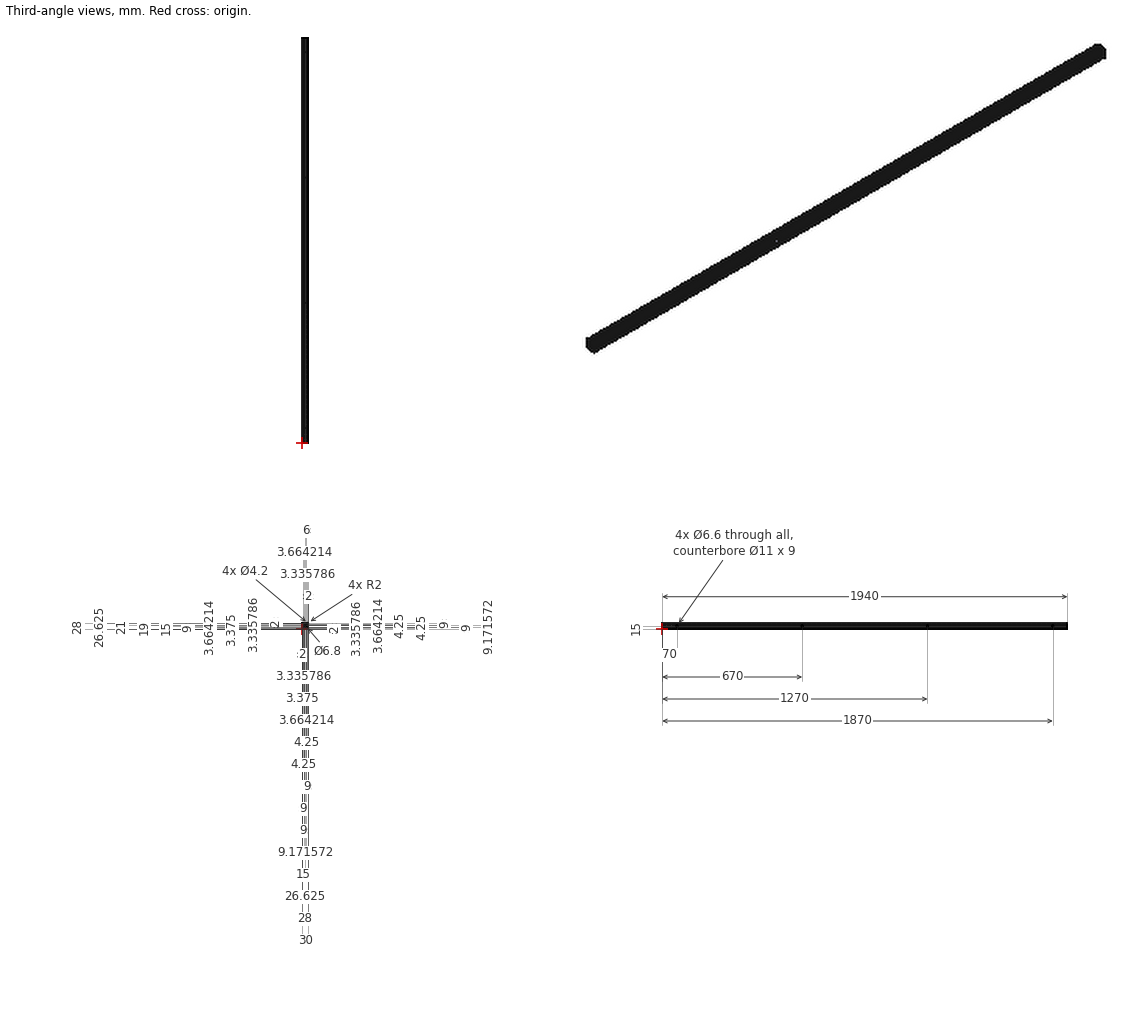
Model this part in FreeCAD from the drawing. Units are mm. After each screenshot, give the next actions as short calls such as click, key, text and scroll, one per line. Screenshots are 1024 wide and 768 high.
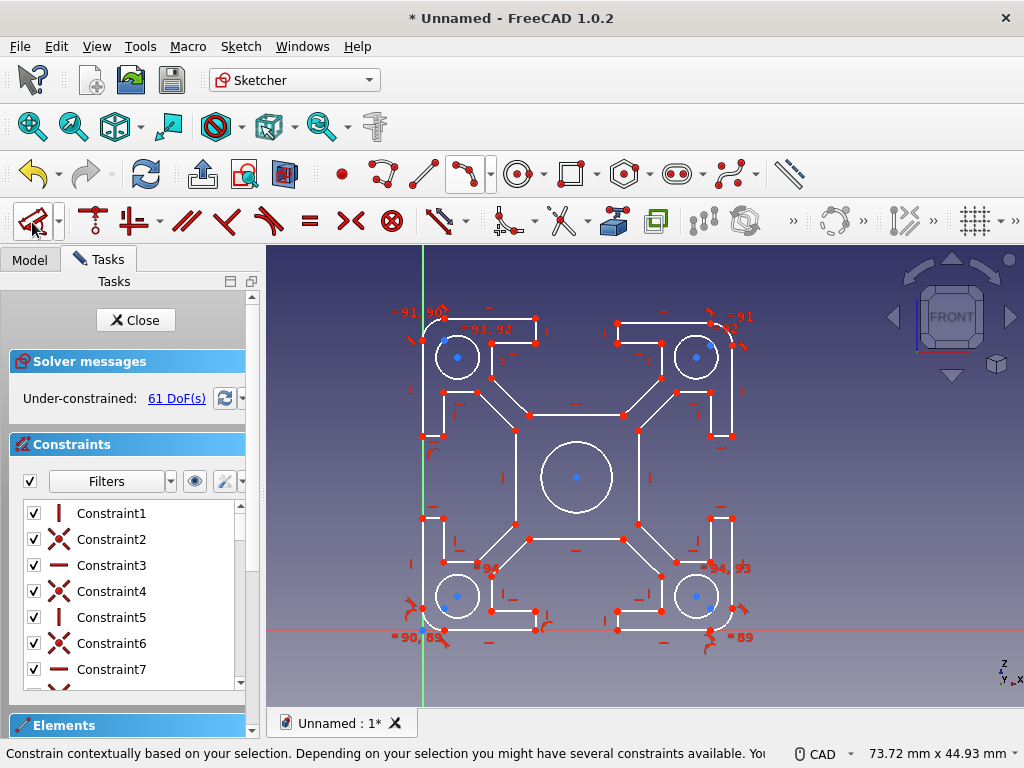
scroll(721, 628, up, 4)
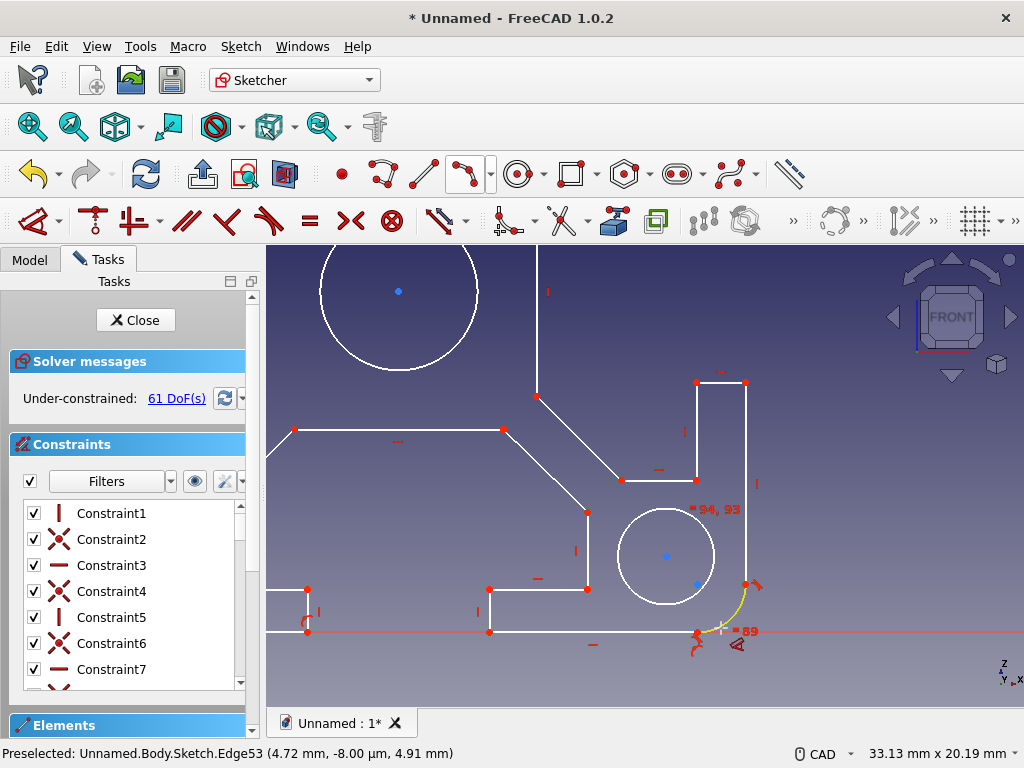
click(719, 627)
click(733, 656)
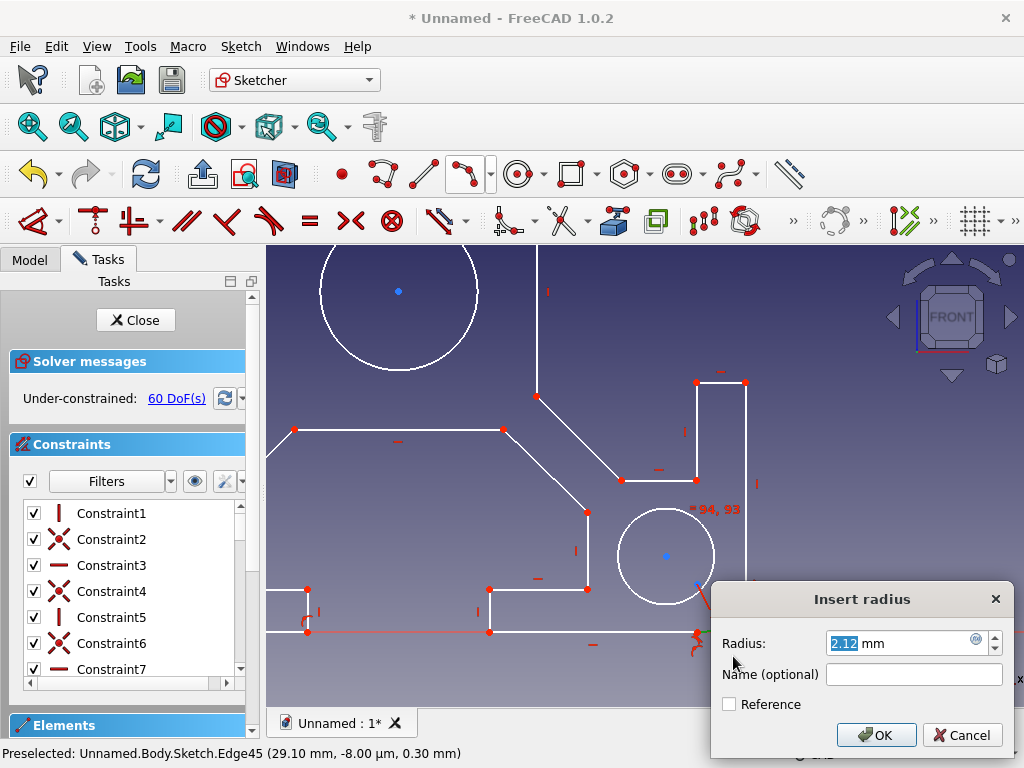
text(2)
key(Return)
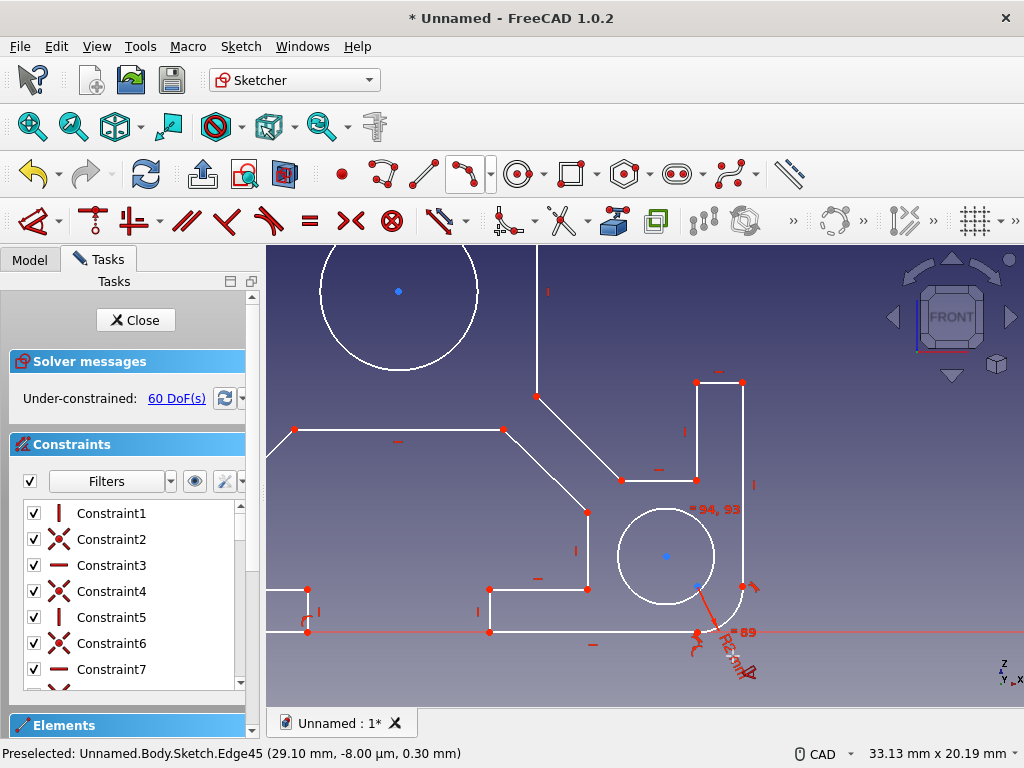
scroll(721, 628, down, 4)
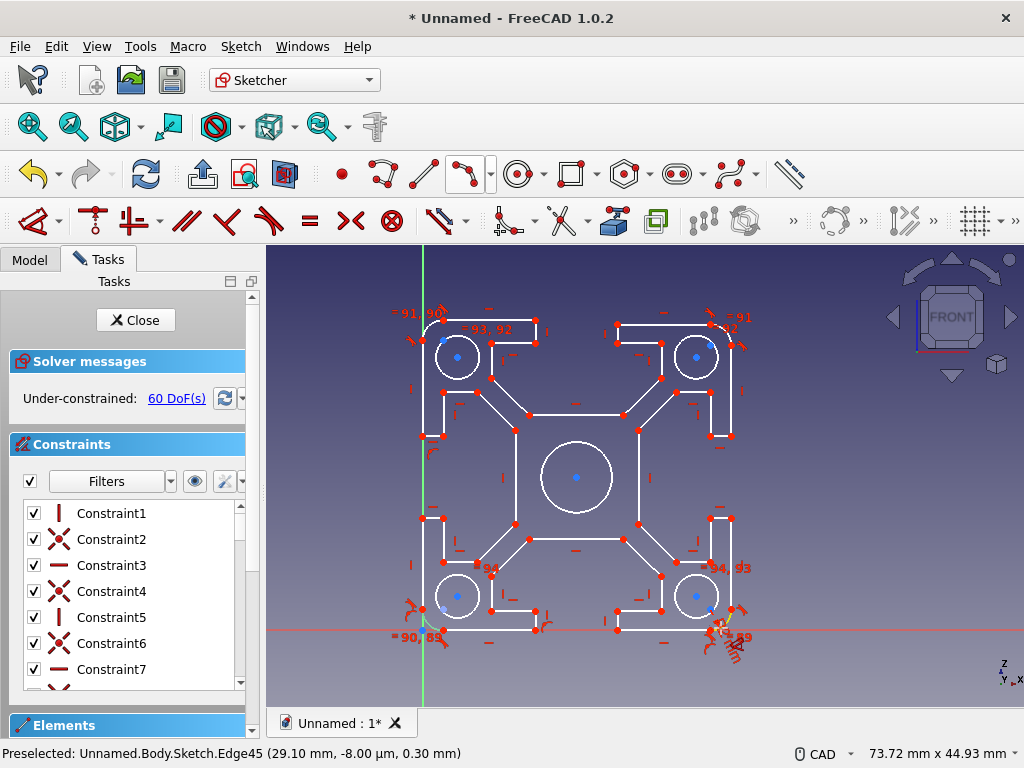
click(681, 342)
click(681, 306)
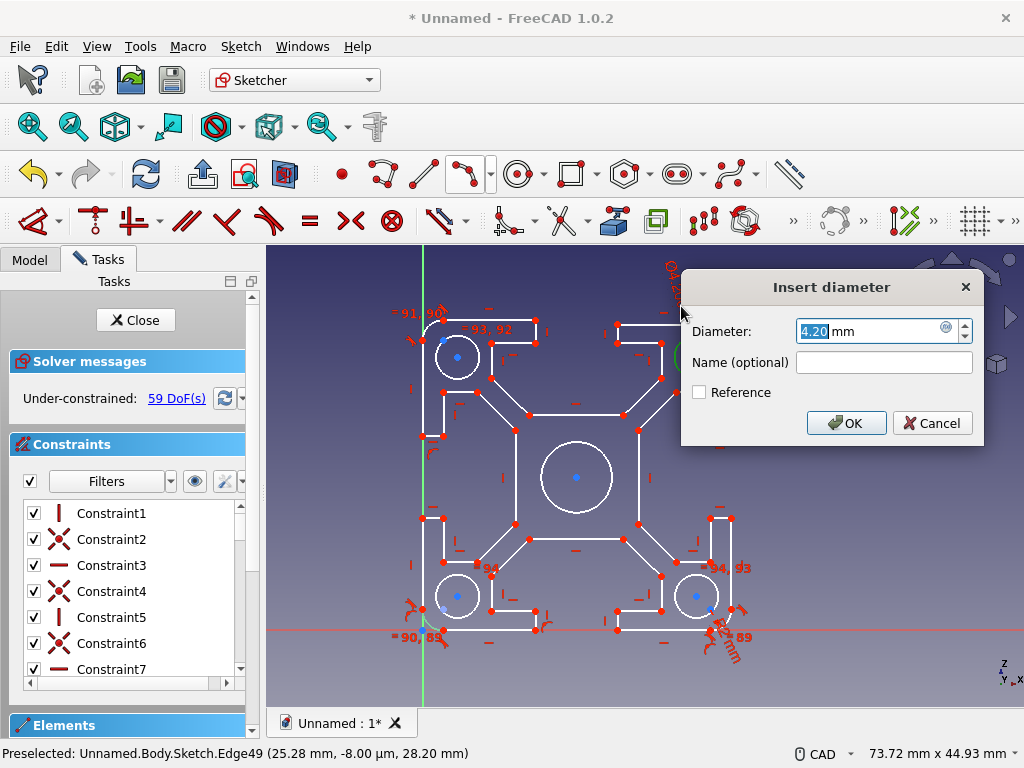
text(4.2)
key(Return)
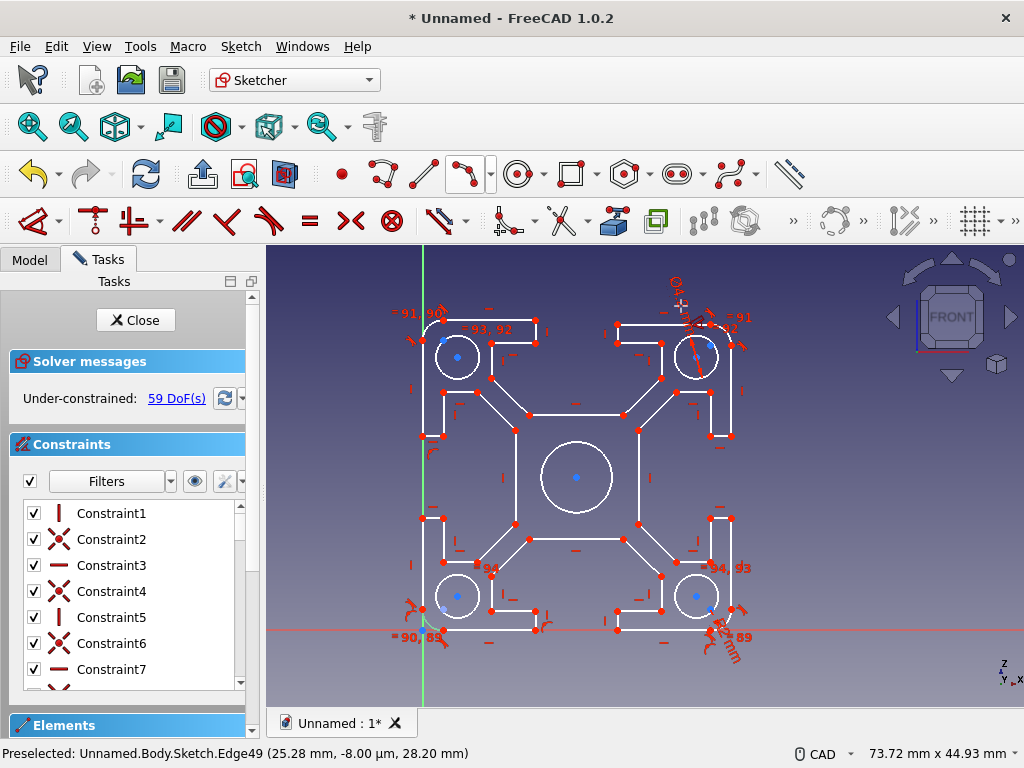
click(602, 452)
click(625, 429)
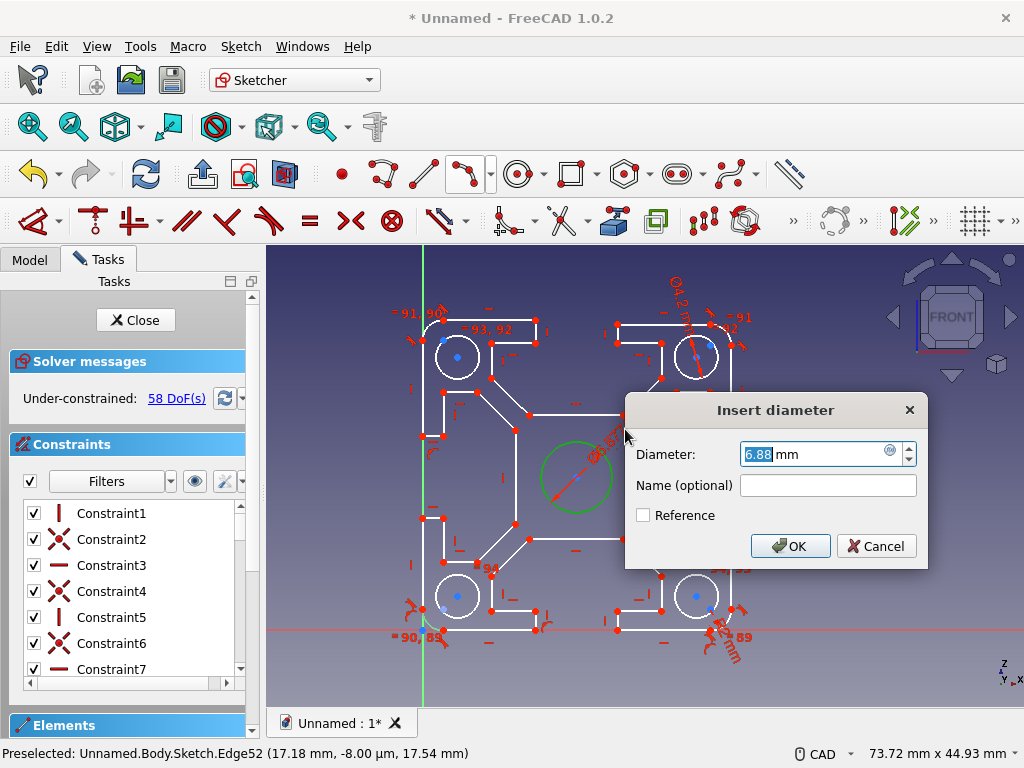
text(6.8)
key(Return)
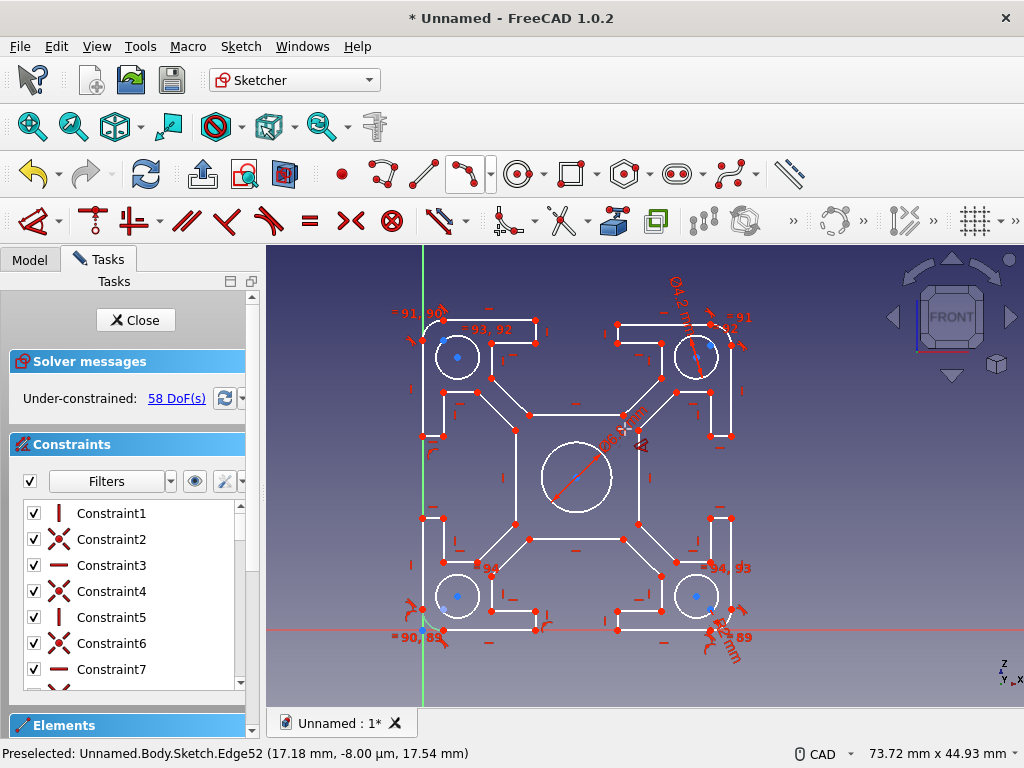
click(731, 372)
click(765, 391)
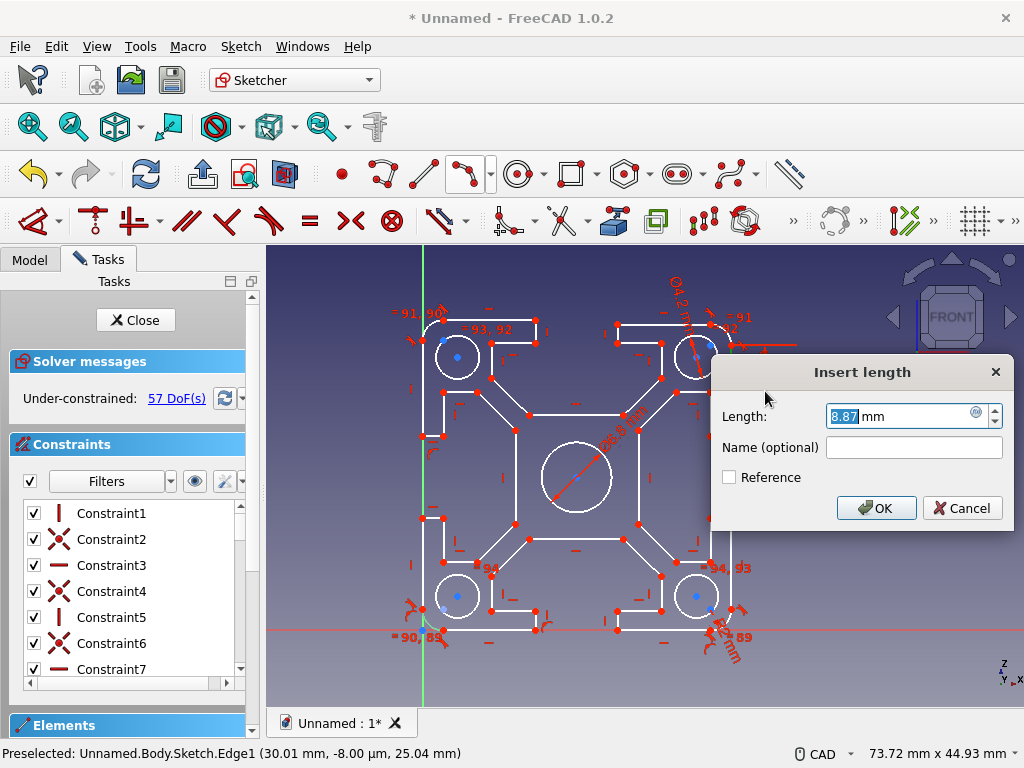
text(9)
key(Return)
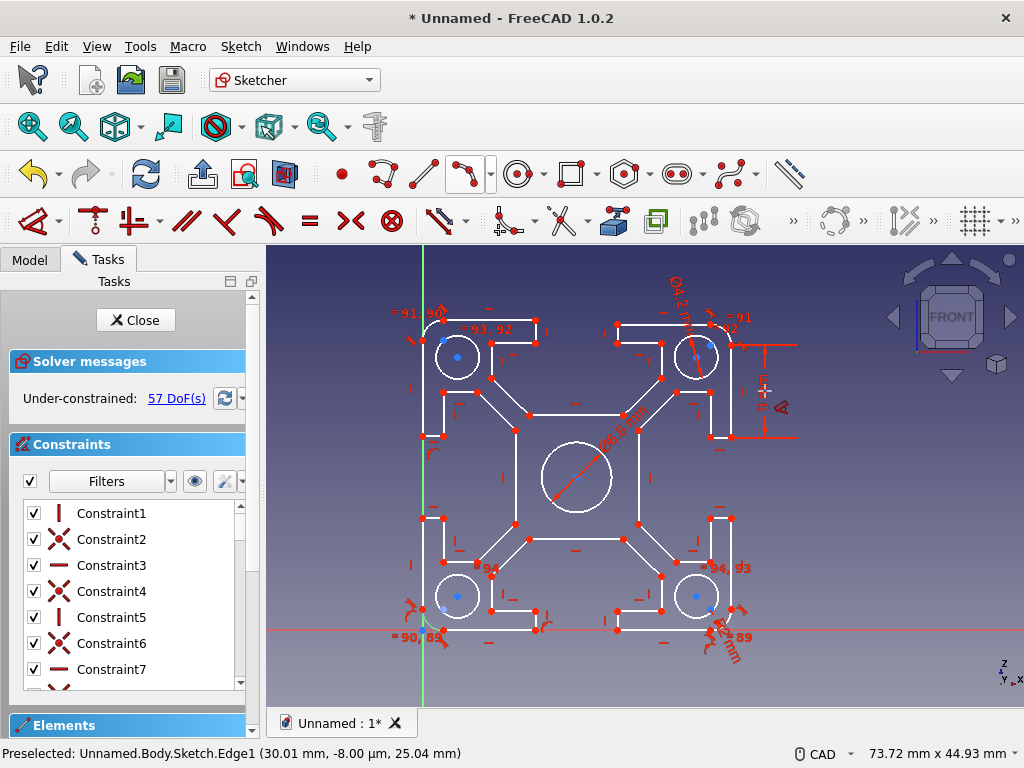
scroll(721, 438, up, 4)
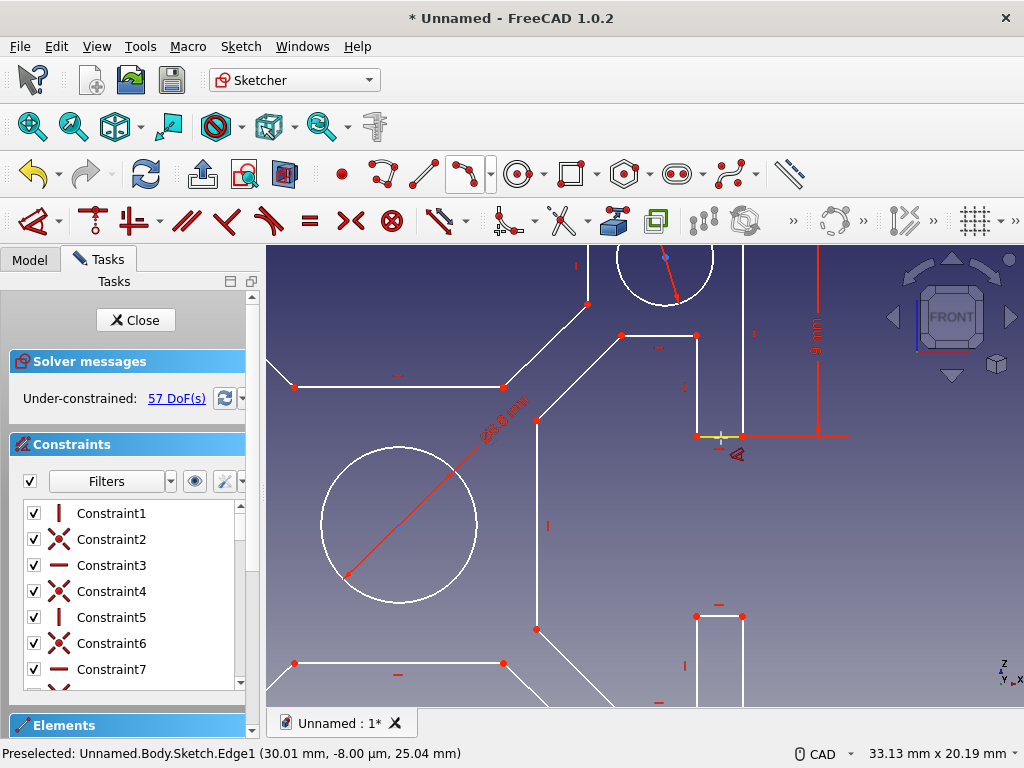
click(720, 437)
click(720, 403)